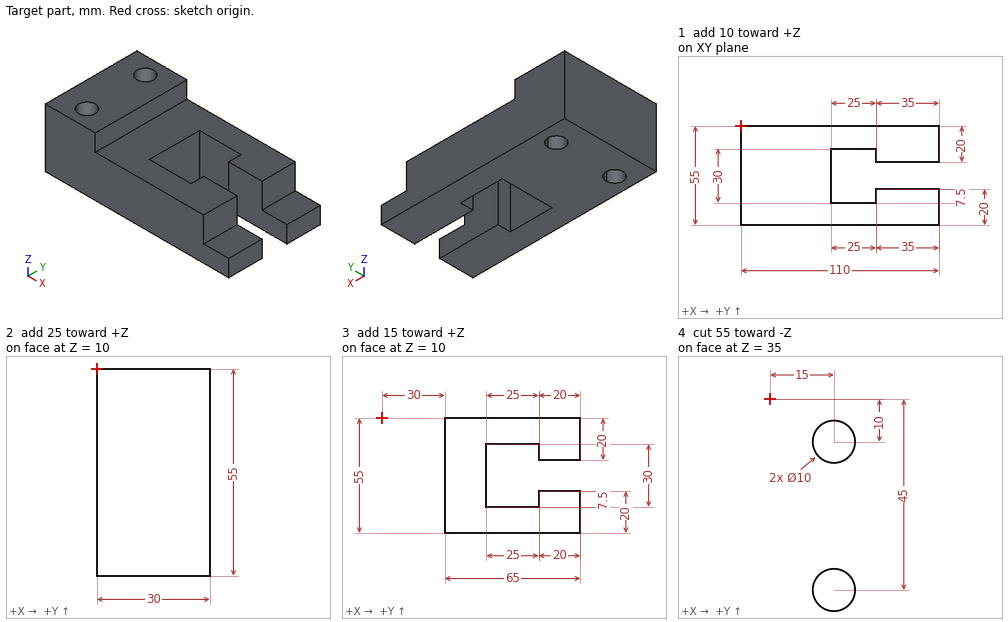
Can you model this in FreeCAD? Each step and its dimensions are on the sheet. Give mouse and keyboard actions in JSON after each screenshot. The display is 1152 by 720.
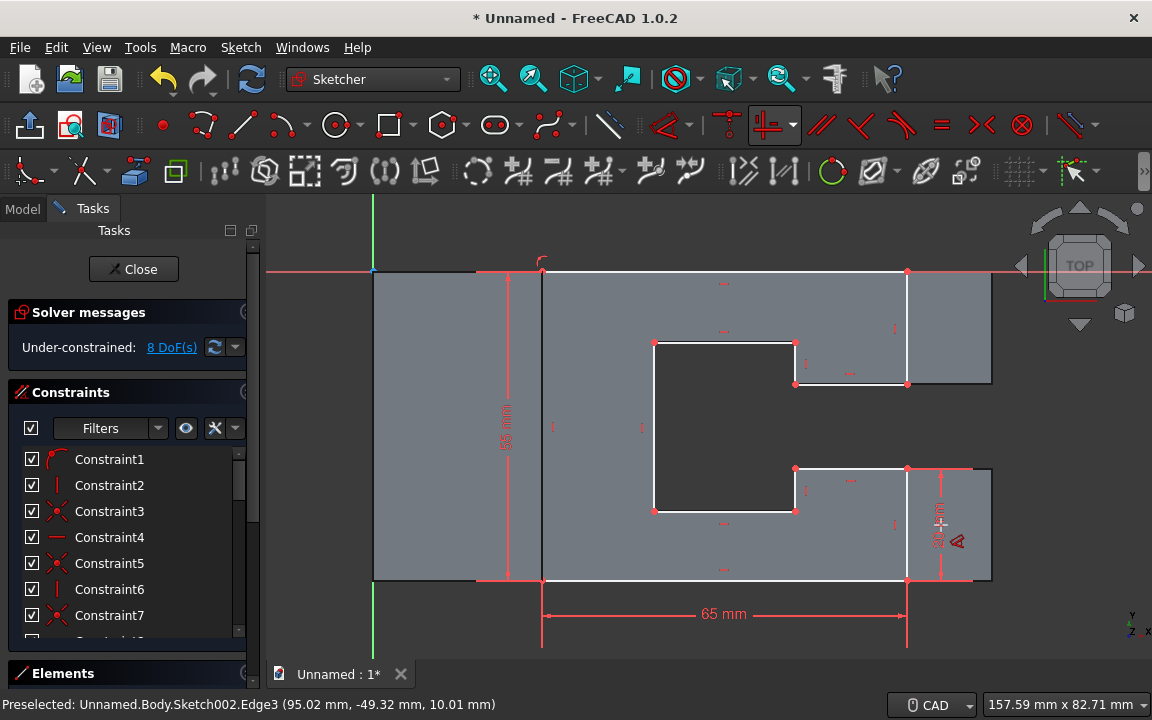
{"action": "left_click", "coordinate": [874, 469]}
{"action": "left_click", "coordinate": [851, 503]}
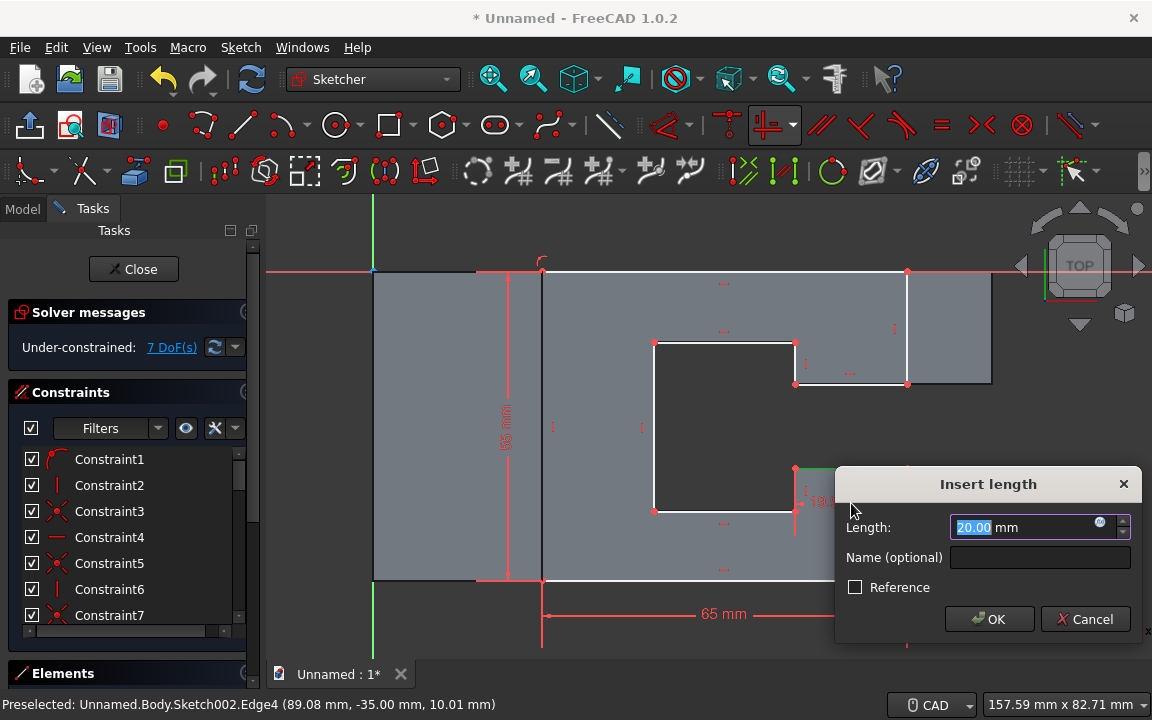
{"action": "type", "text": "20"}
{"action": "key", "text": "Return"}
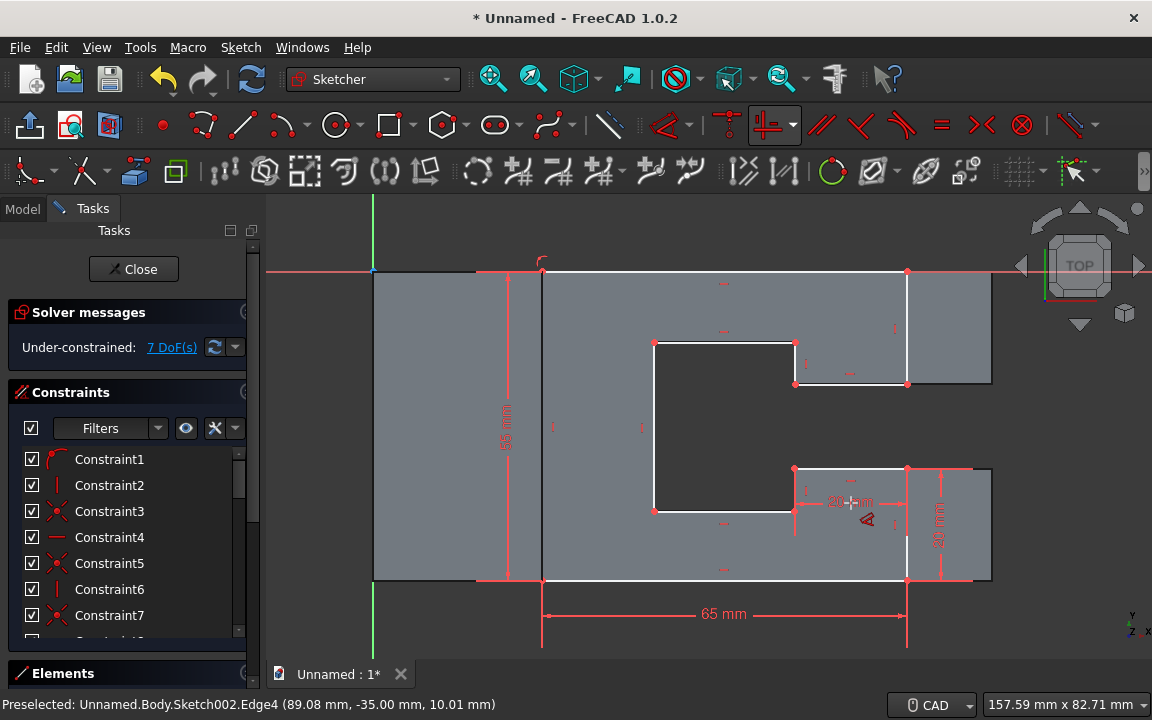
{"action": "left_click", "coordinate": [753, 512]}
{"action": "left_click", "coordinate": [724, 546]}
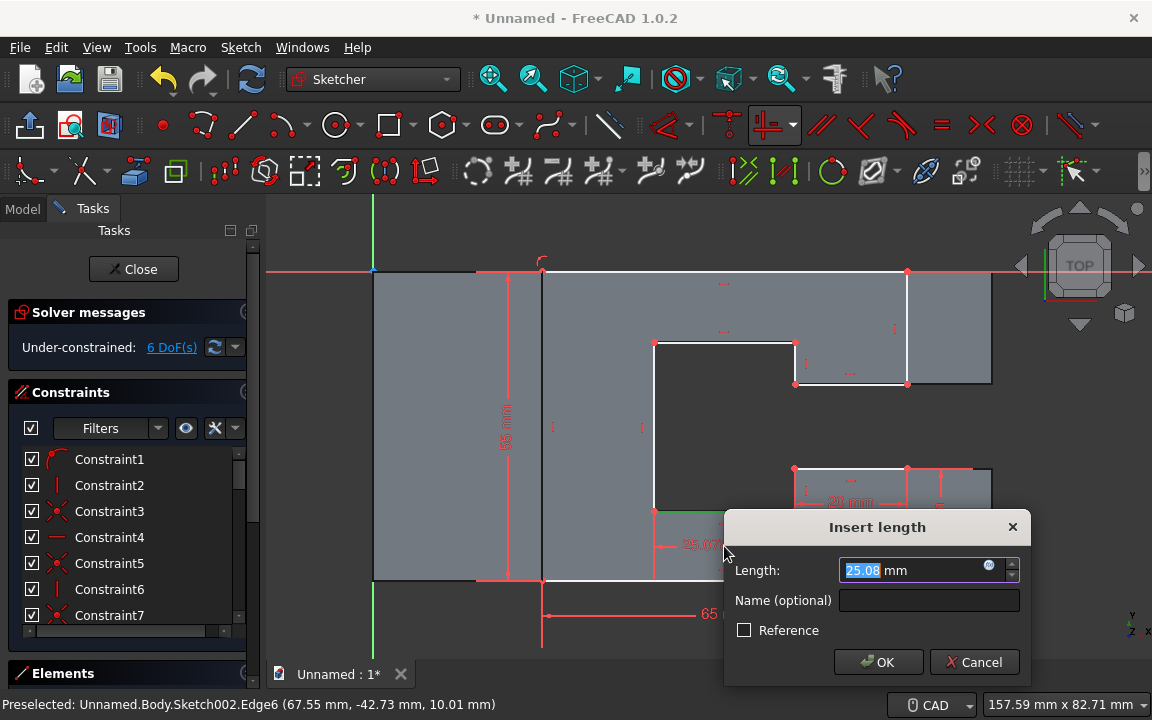
{"action": "type", "text": "25"}
{"action": "key", "text": "Return"}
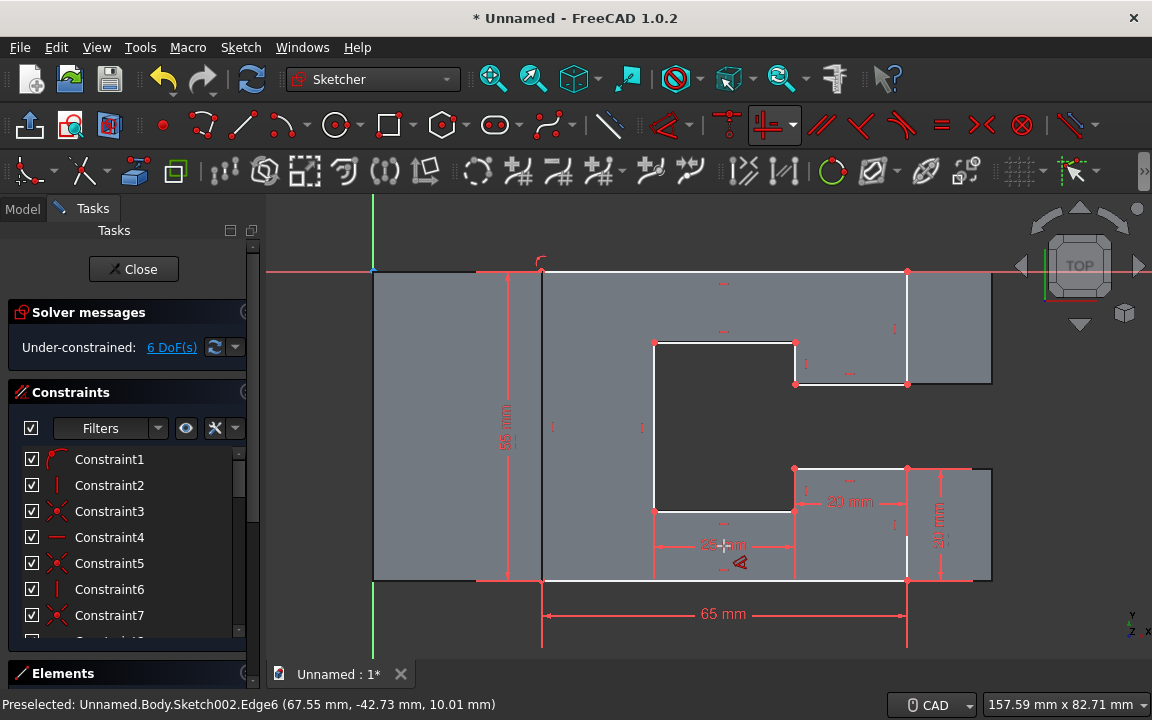
{"action": "left_click", "coordinate": [654, 461]}
{"action": "left_click", "coordinate": [688, 428]}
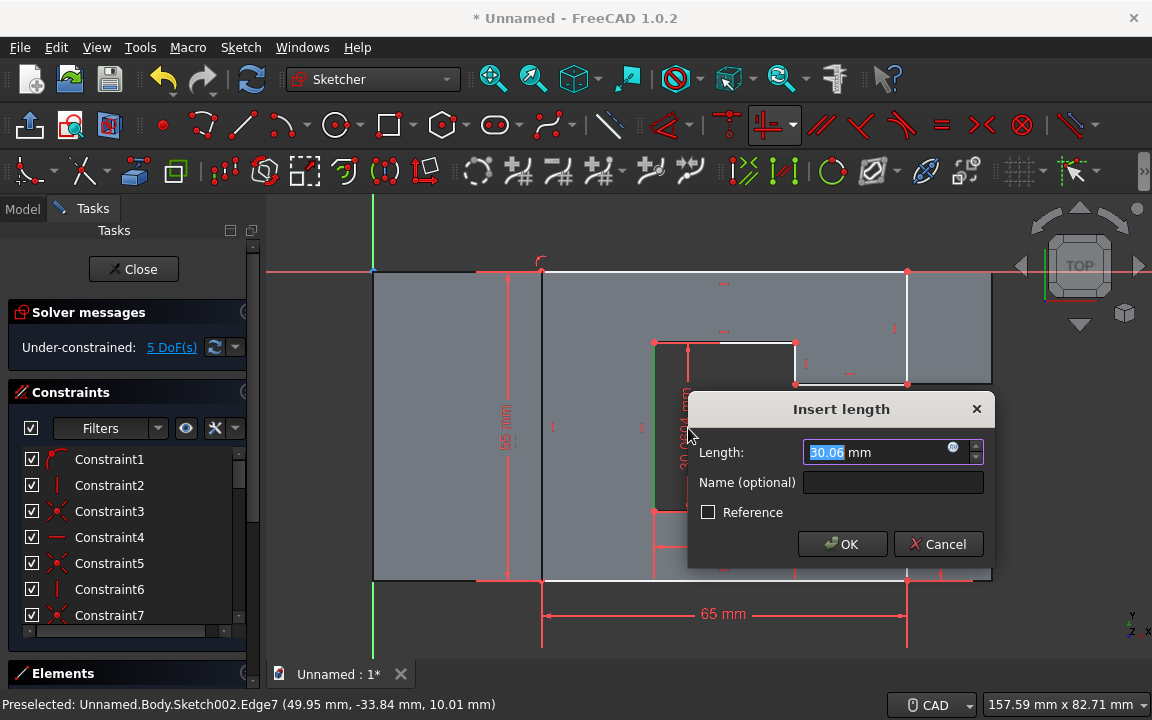
{"action": "type", "text": "30"}
{"action": "key", "text": "Return"}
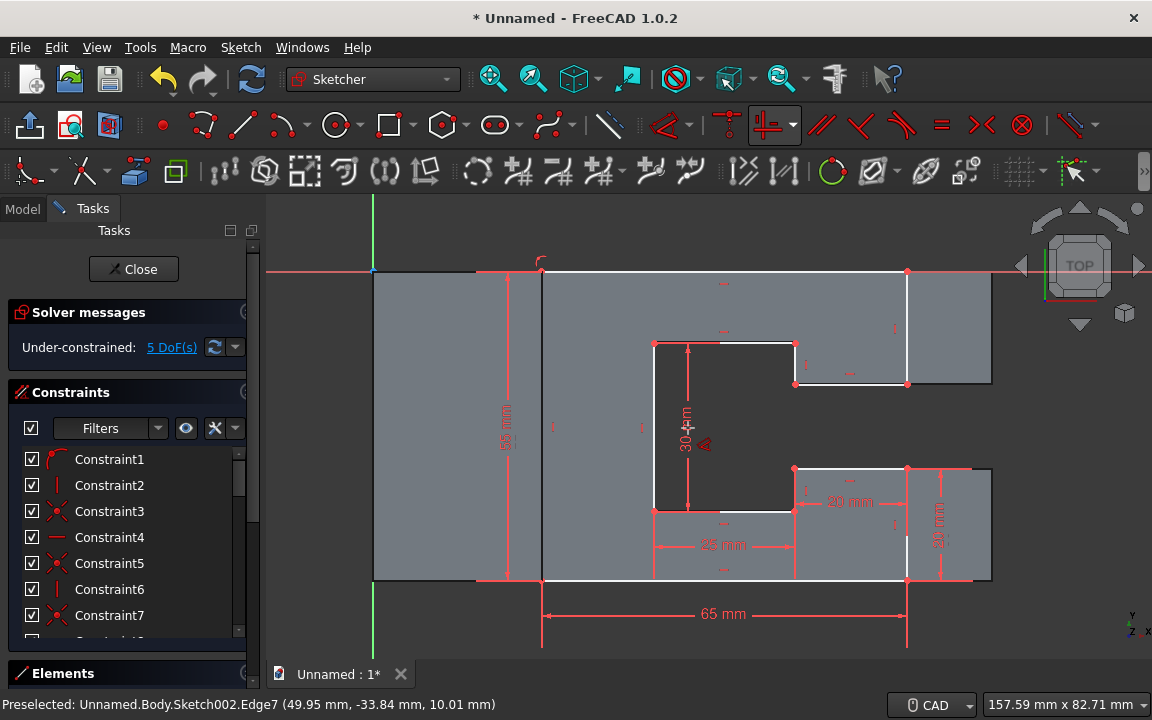
{"action": "left_click", "coordinate": [696, 343]}
{"action": "left_click", "coordinate": [725, 309]}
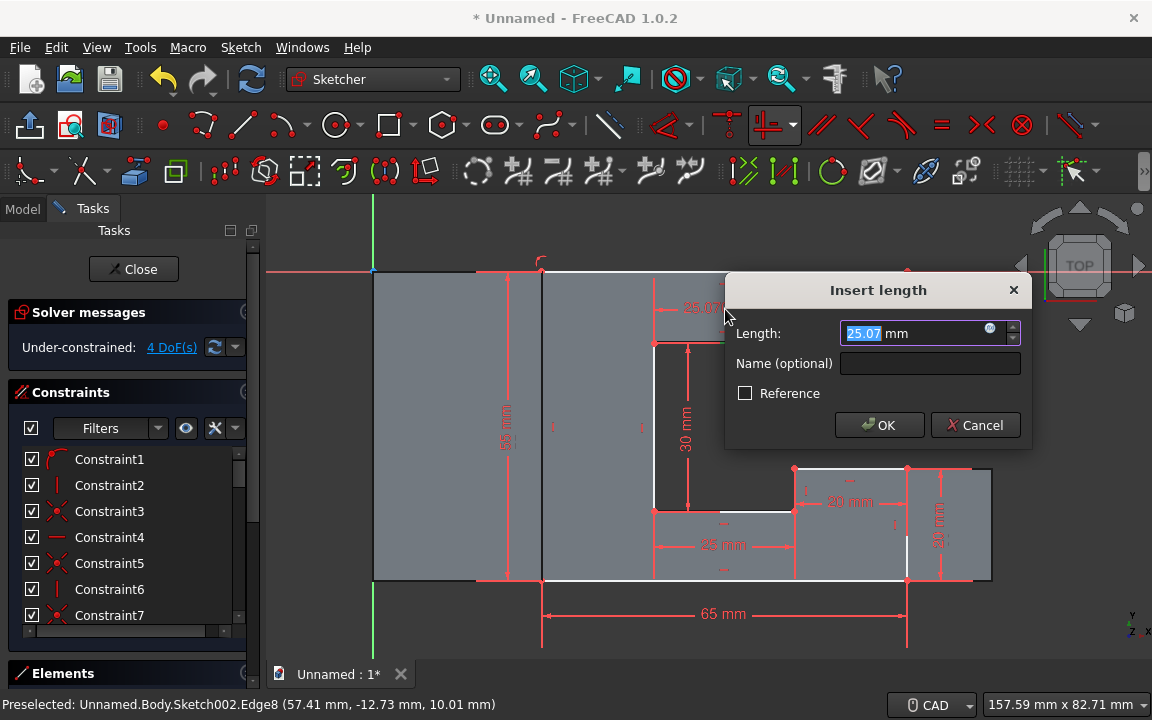
{"action": "type", "text": "25"}
{"action": "key", "text": "Return"}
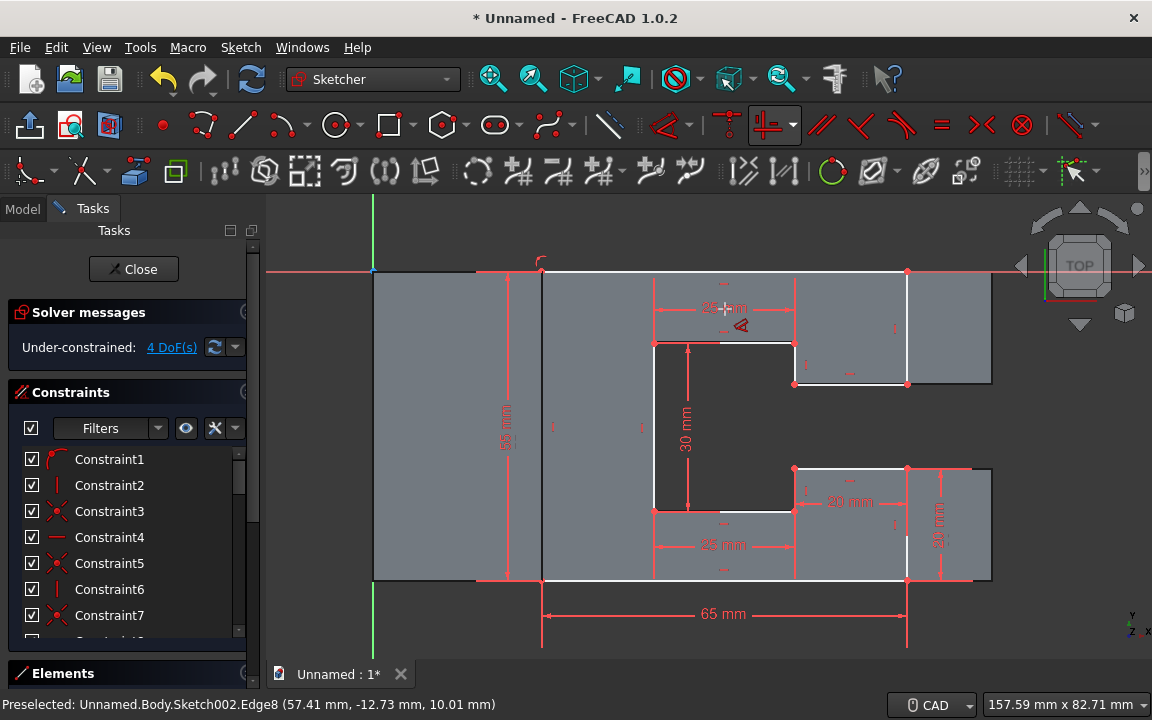
{"action": "left_click", "coordinate": [828, 385]}
{"action": "left_click", "coordinate": [851, 351]}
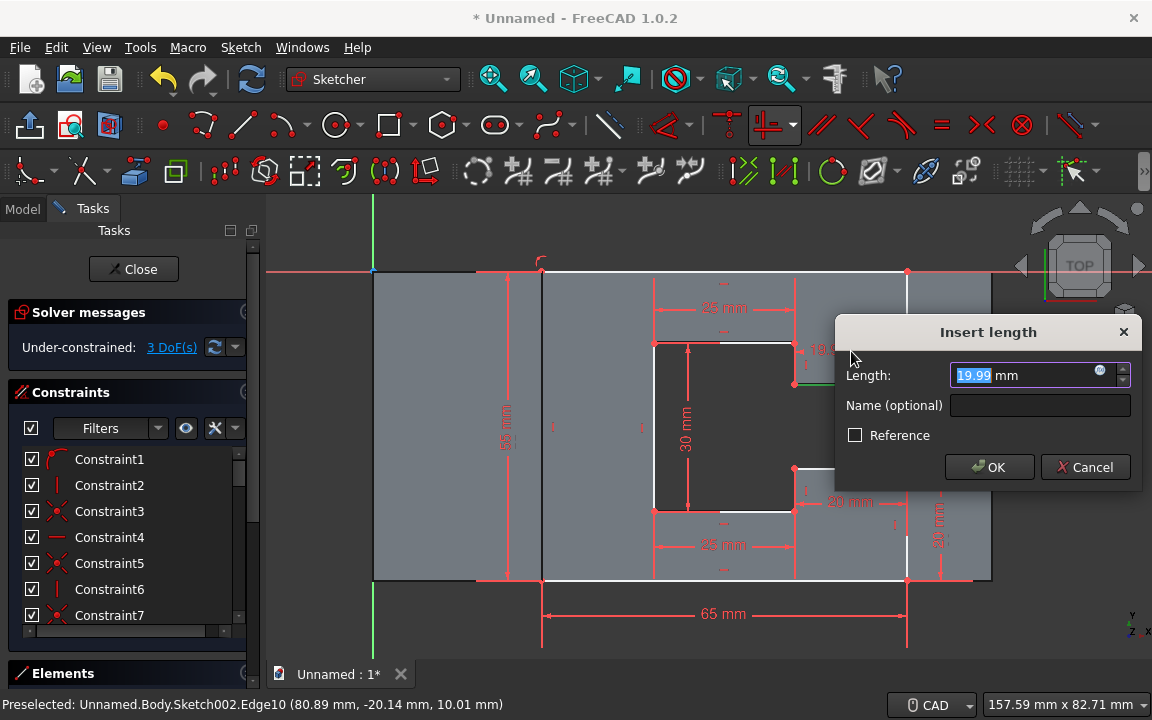
{"action": "type", "text": "20"}
{"action": "key", "text": "Return"}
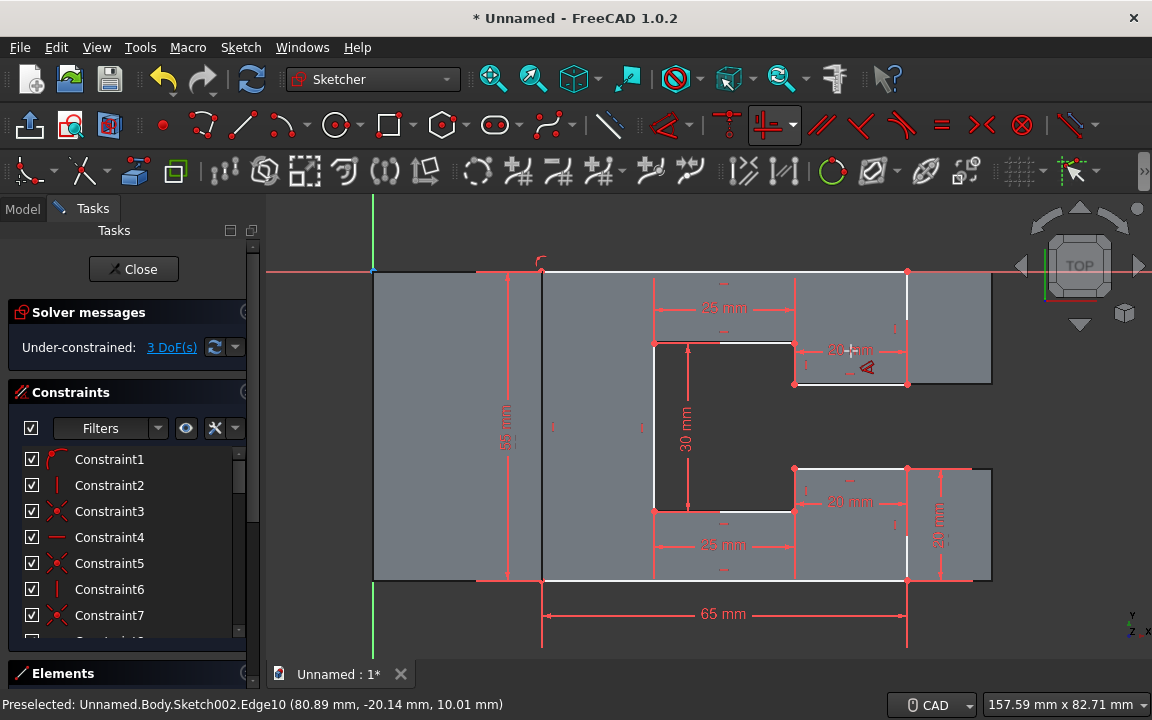
{"action": "left_click", "coordinate": [907, 351]}
{"action": "left_click", "coordinate": [941, 328]}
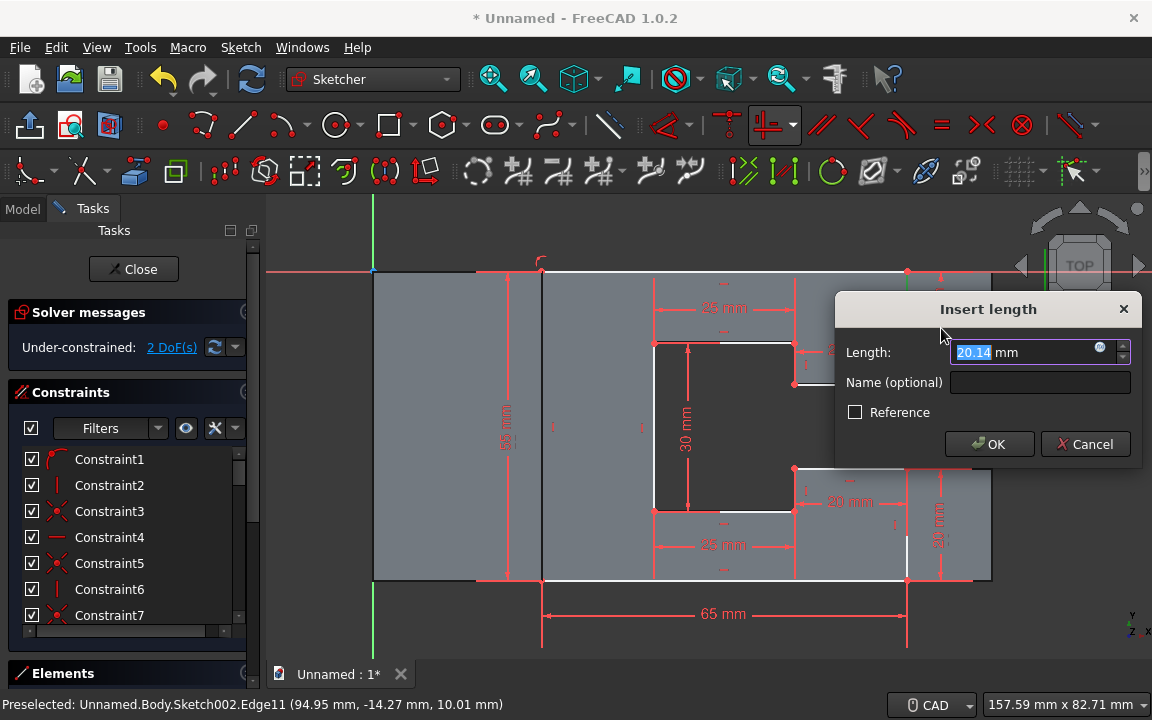
{"action": "type", "text": "20"}
{"action": "key", "text": "Return"}